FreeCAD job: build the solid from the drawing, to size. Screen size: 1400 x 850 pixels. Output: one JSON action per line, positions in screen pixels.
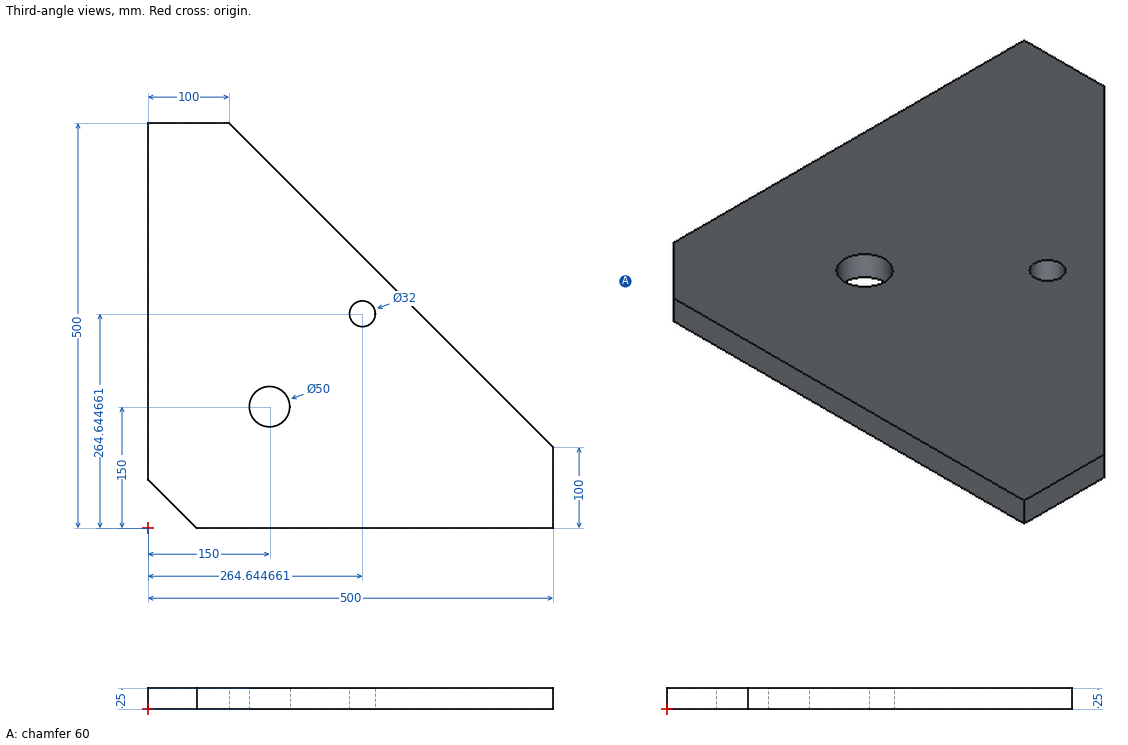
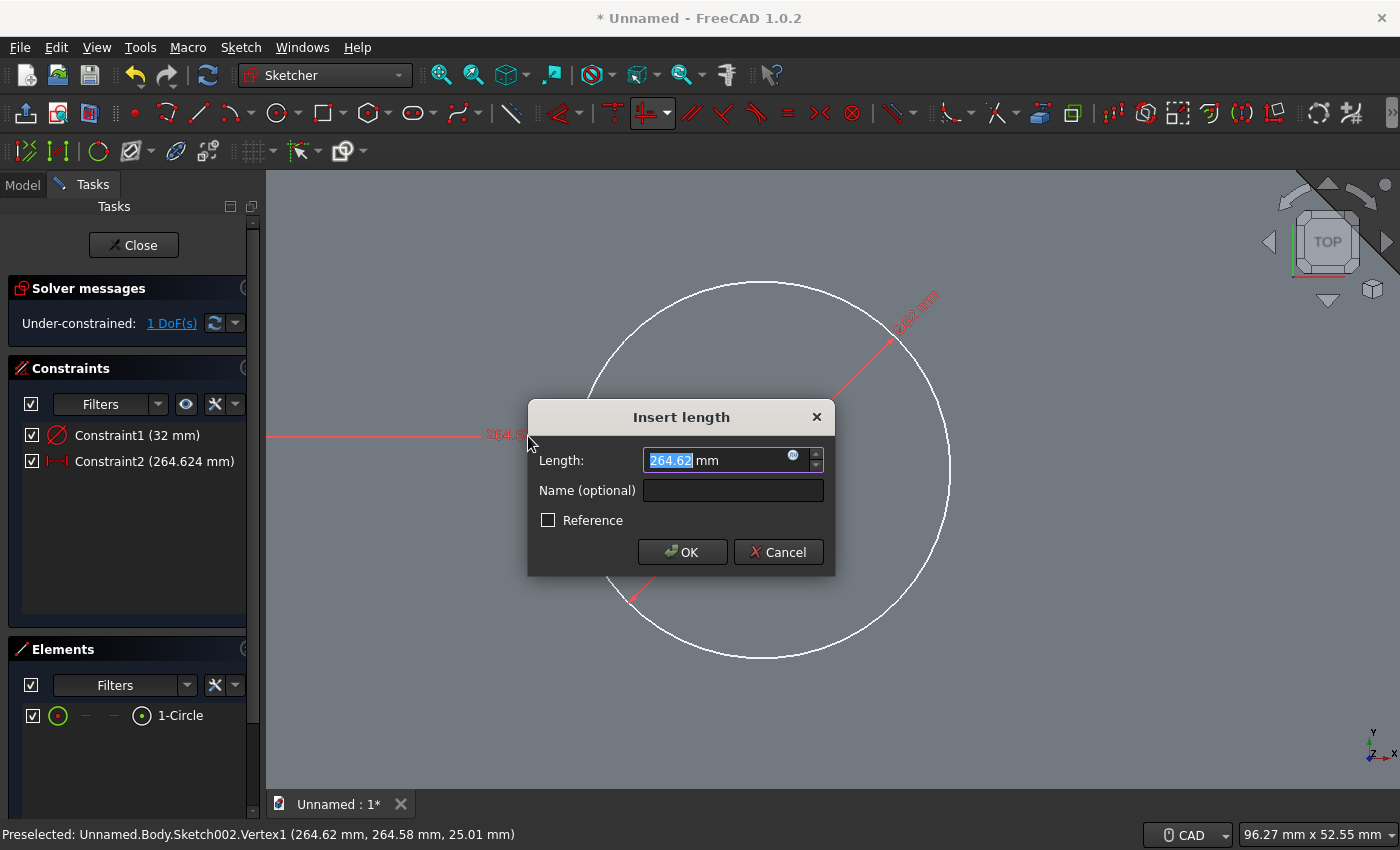
{"action": "type", "text": "264.644661"}
{"action": "key", "text": "Return"}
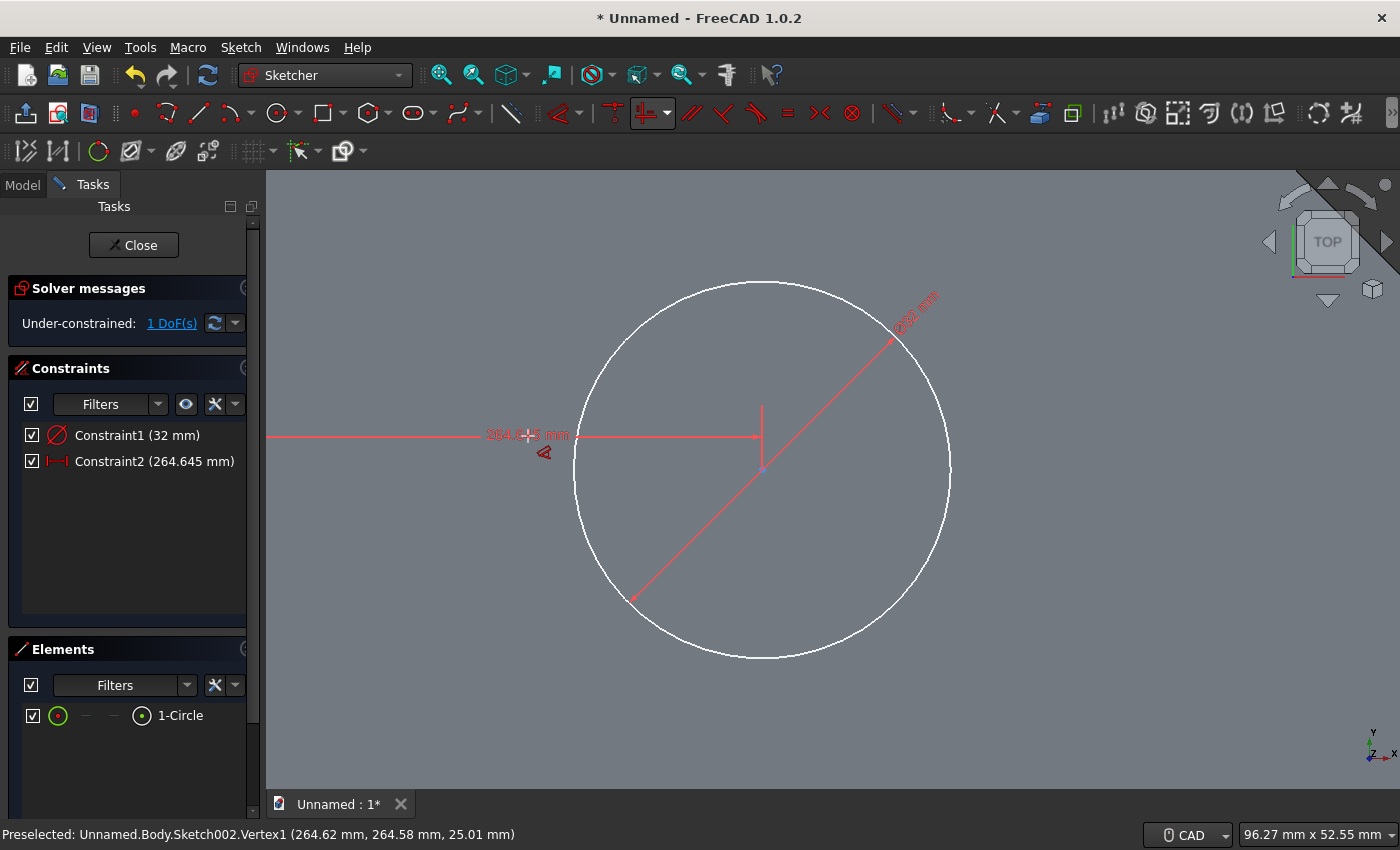
{"action": "left_click", "coordinate": [762, 470]}
{"action": "left_click", "coordinate": [796, 615]}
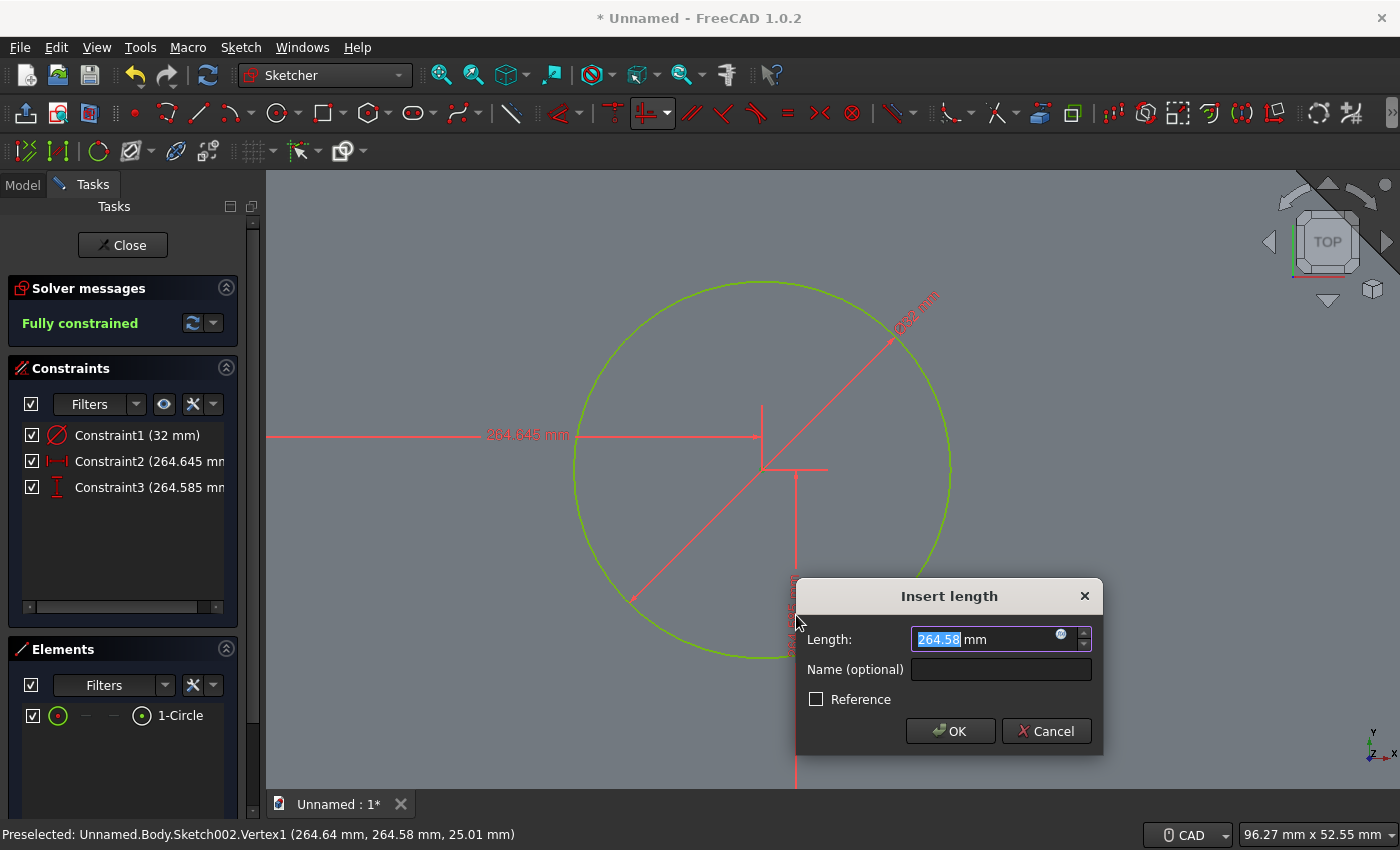
{"action": "type", "text": "264.644661"}
{"action": "key", "text": "Return"}
{"action": "key", "text": "Escape"}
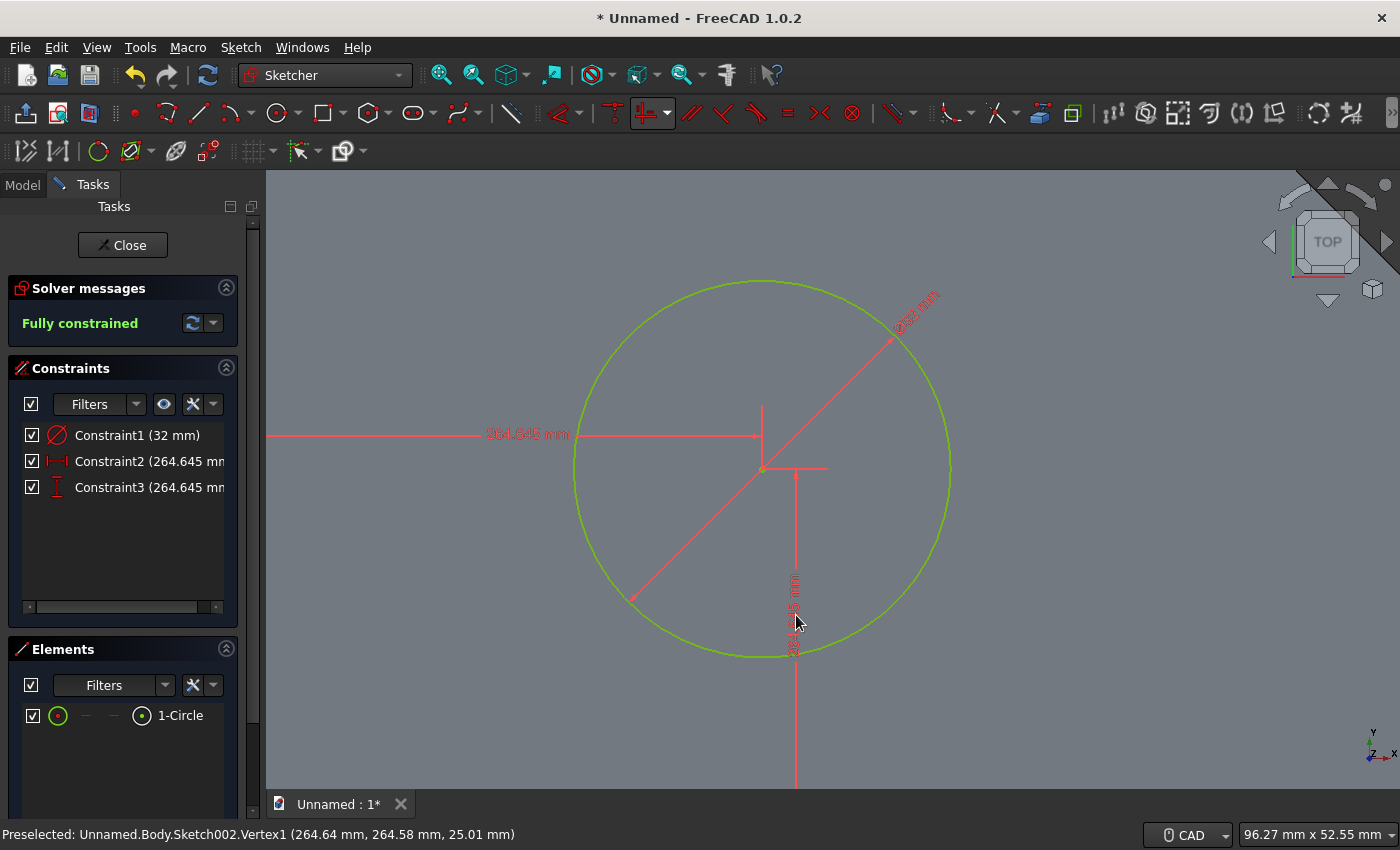
{"action": "left_click", "coordinate": [123, 245]}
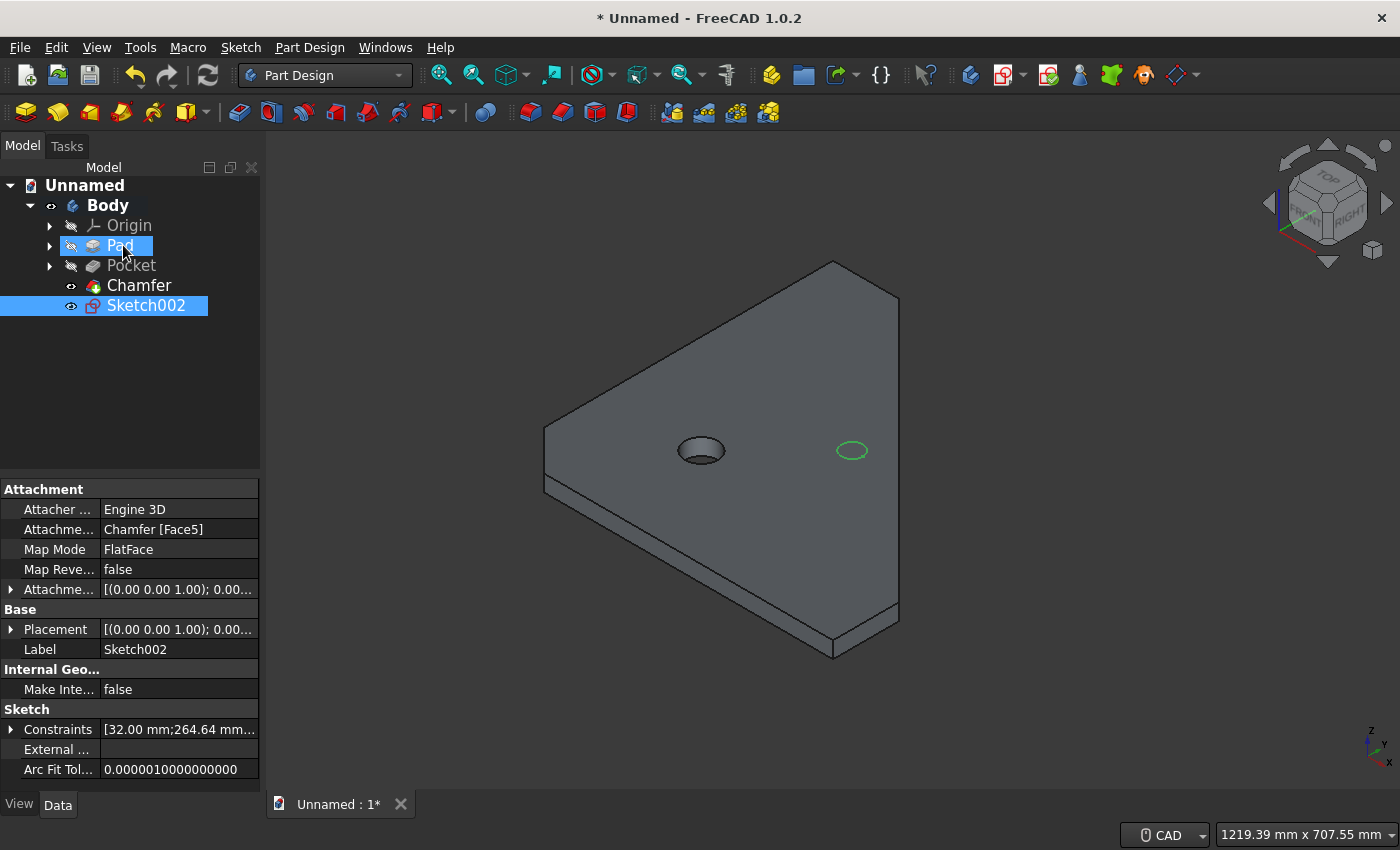
{"action": "left_click", "coordinate": [240, 112]}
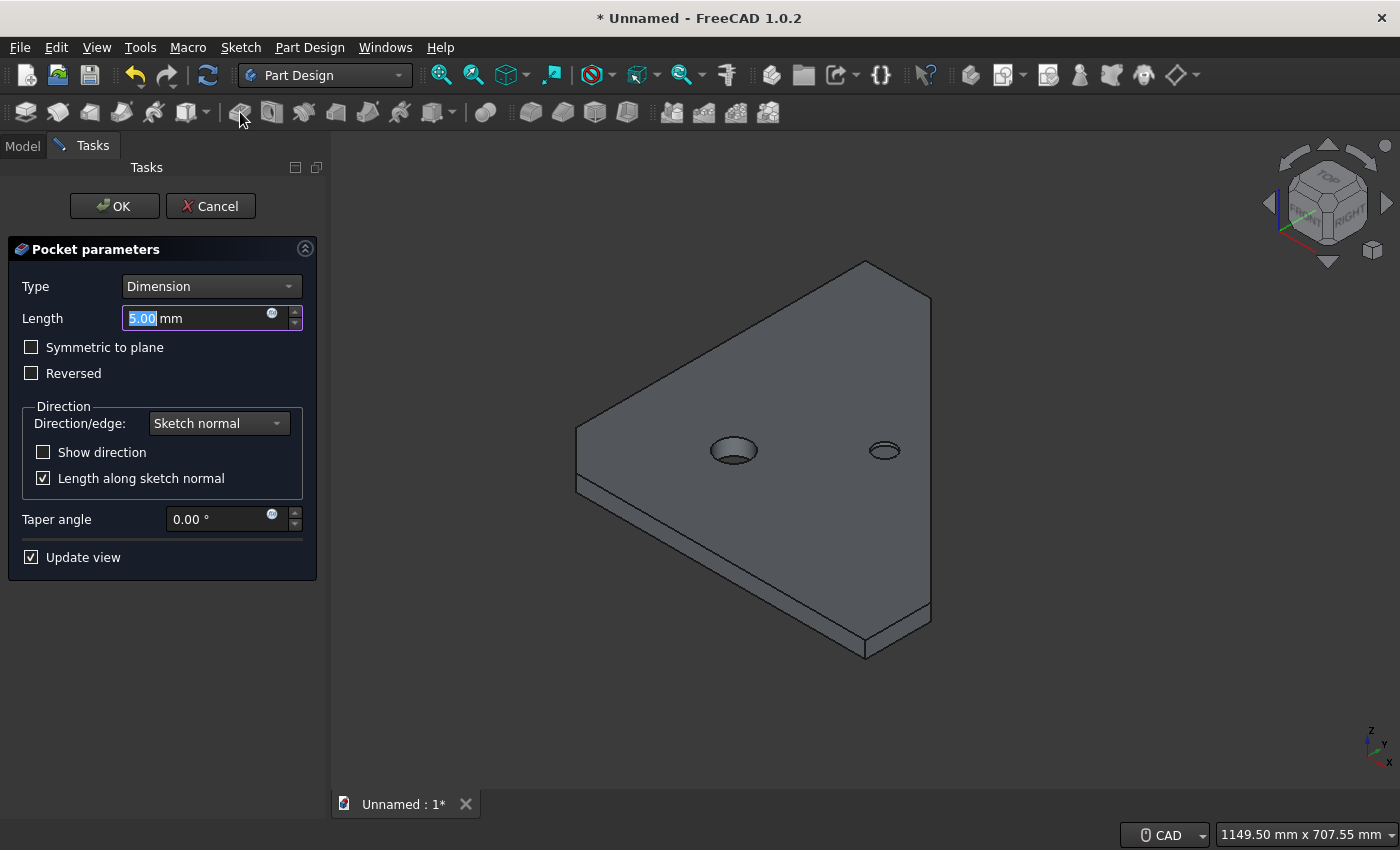
{"action": "left_click", "coordinate": [212, 286]}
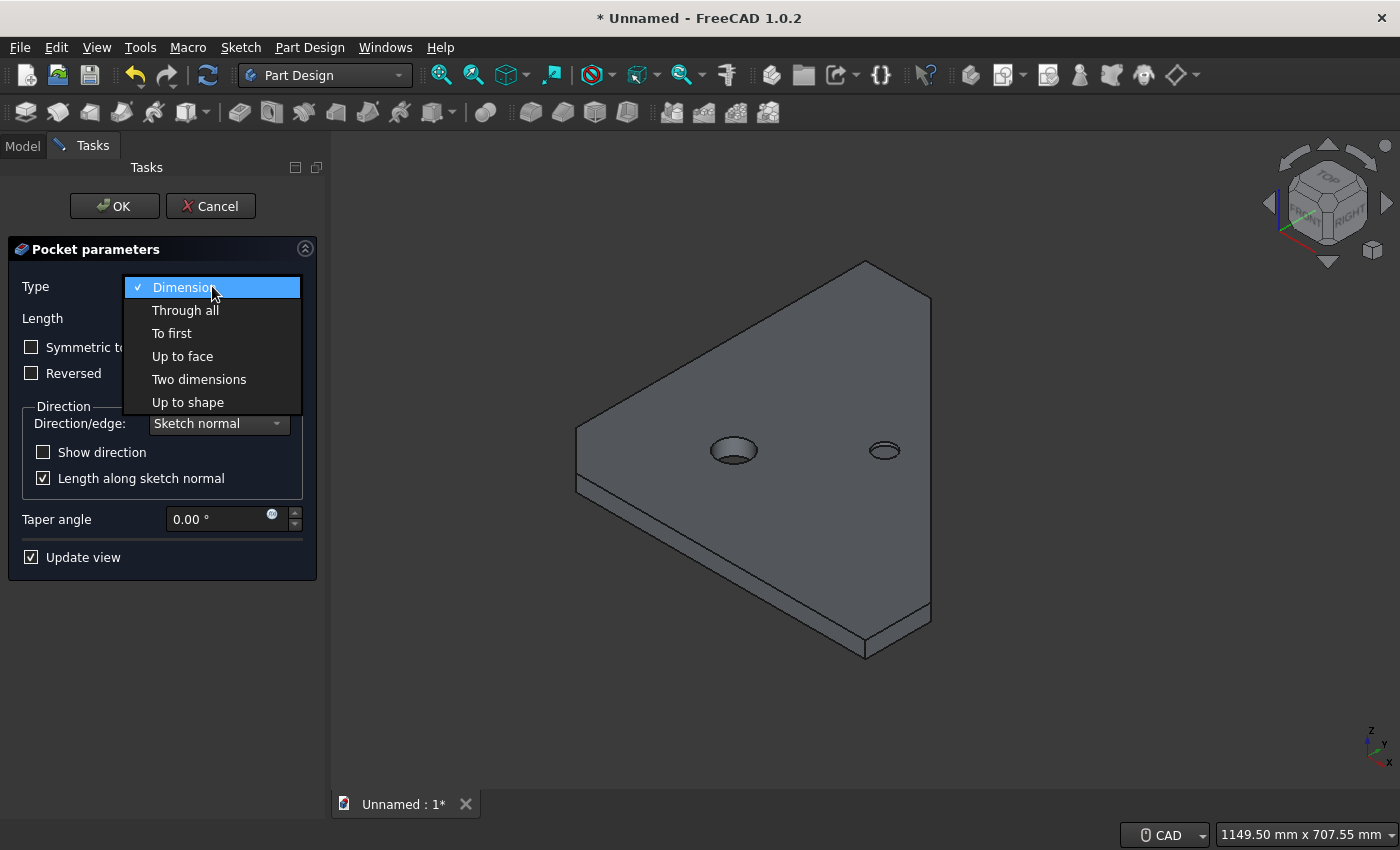
{"action": "left_click", "coordinate": [212, 310]}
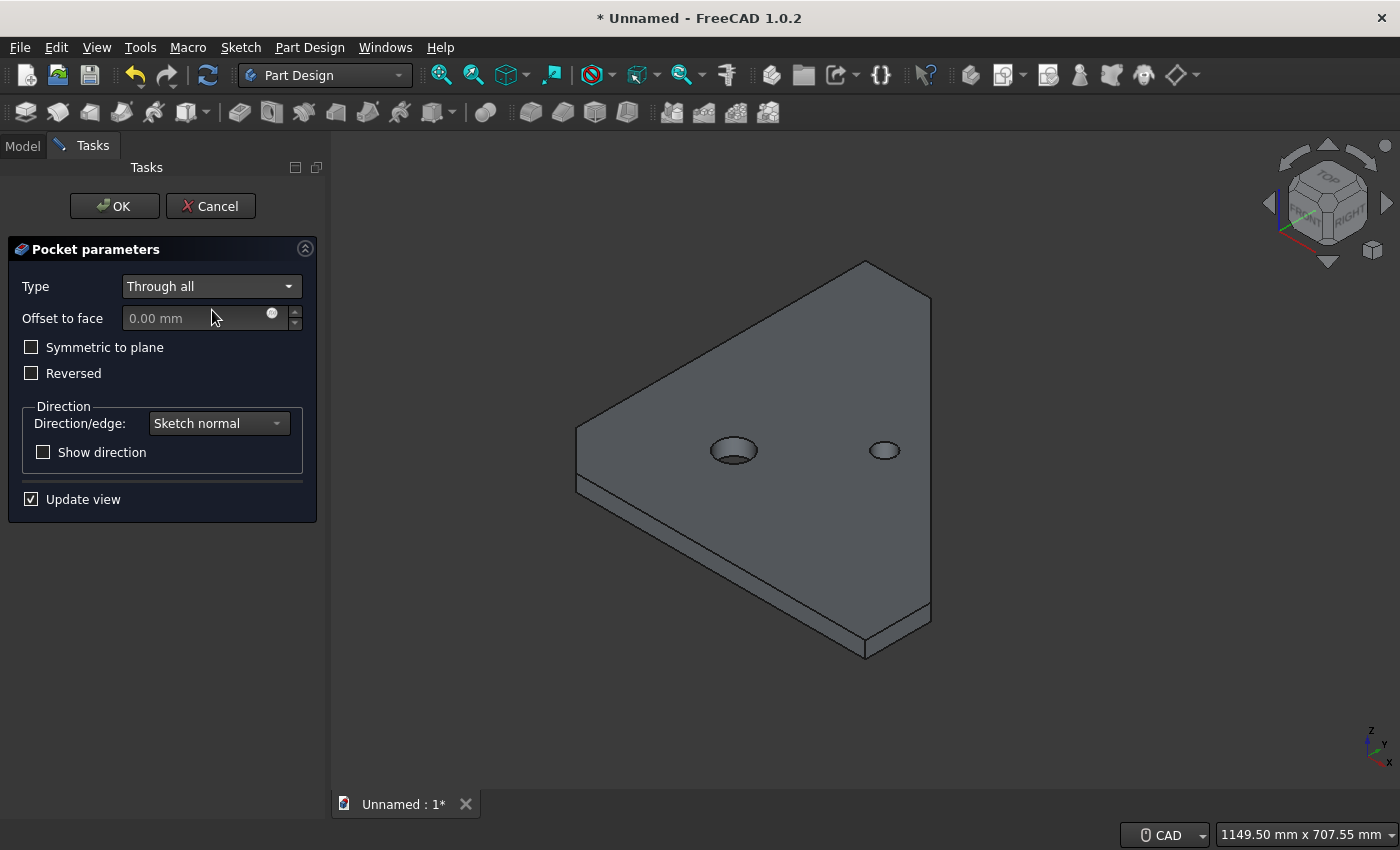
{"action": "left_click", "coordinate": [115, 206]}